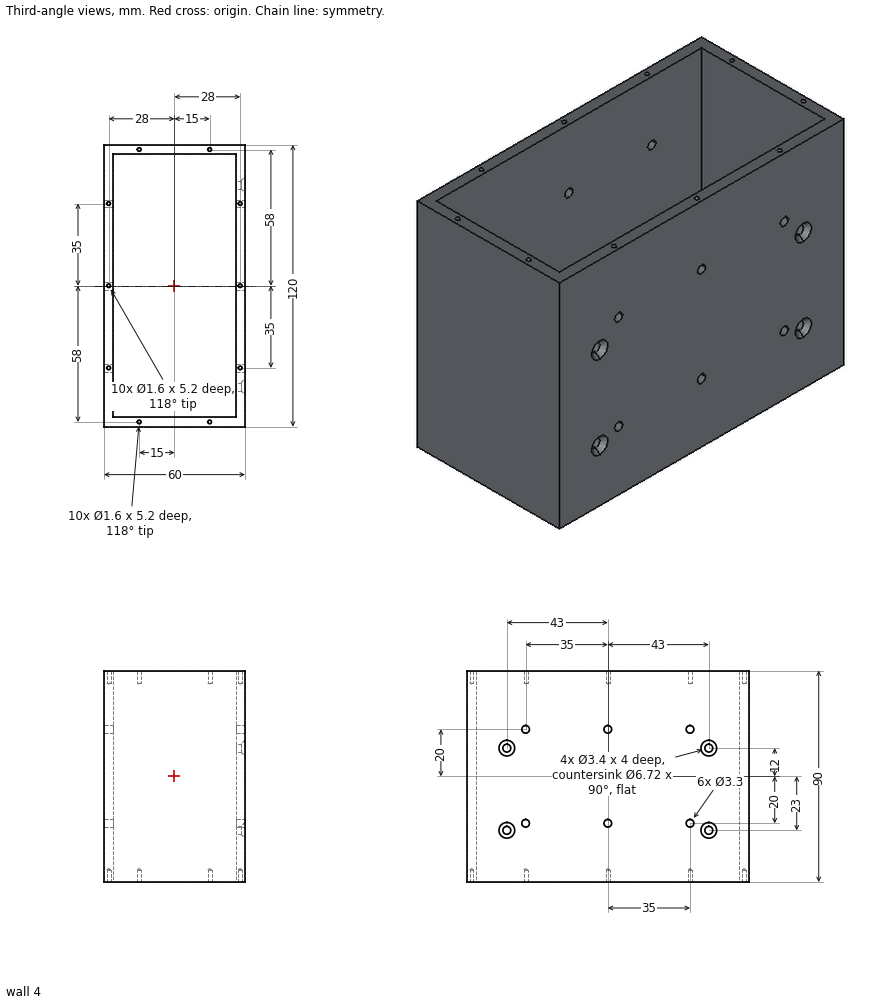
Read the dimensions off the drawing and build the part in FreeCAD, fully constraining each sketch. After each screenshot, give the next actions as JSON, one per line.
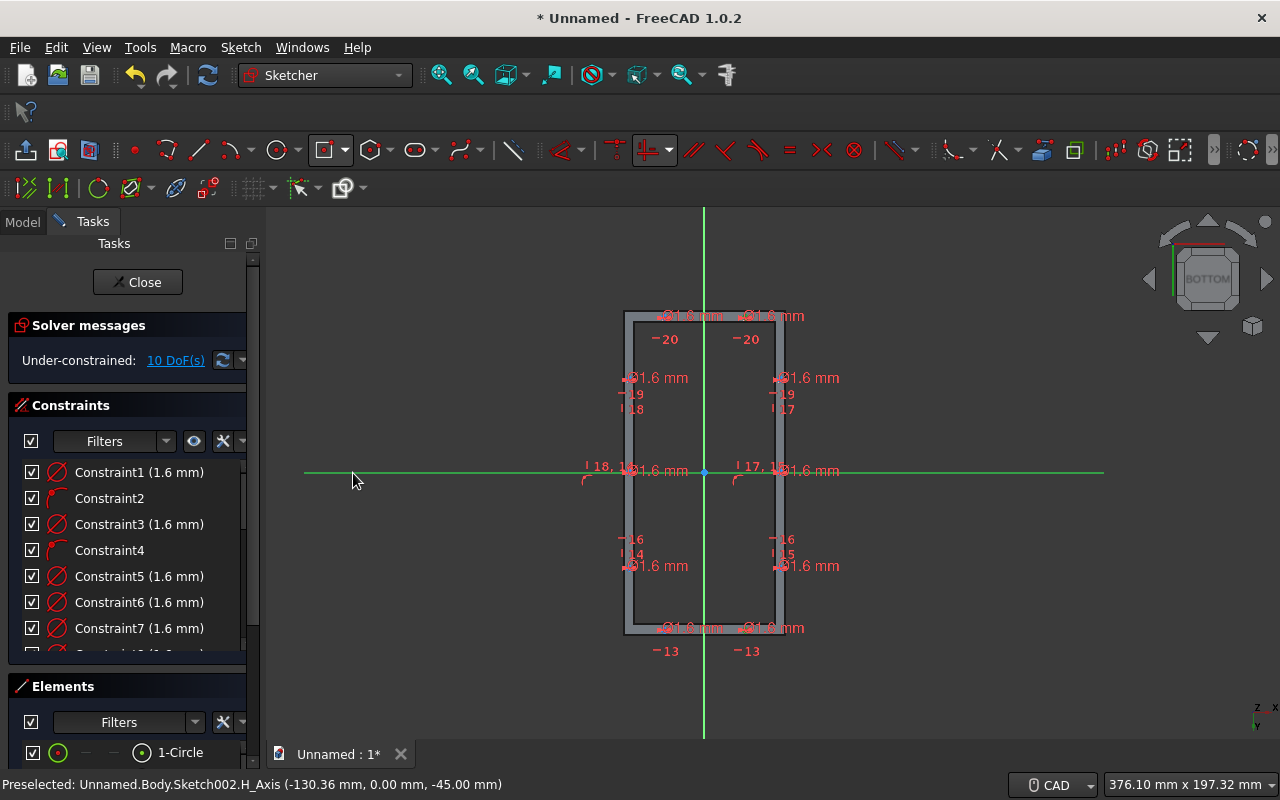
{"action": "left_click", "coordinate": [822, 150]}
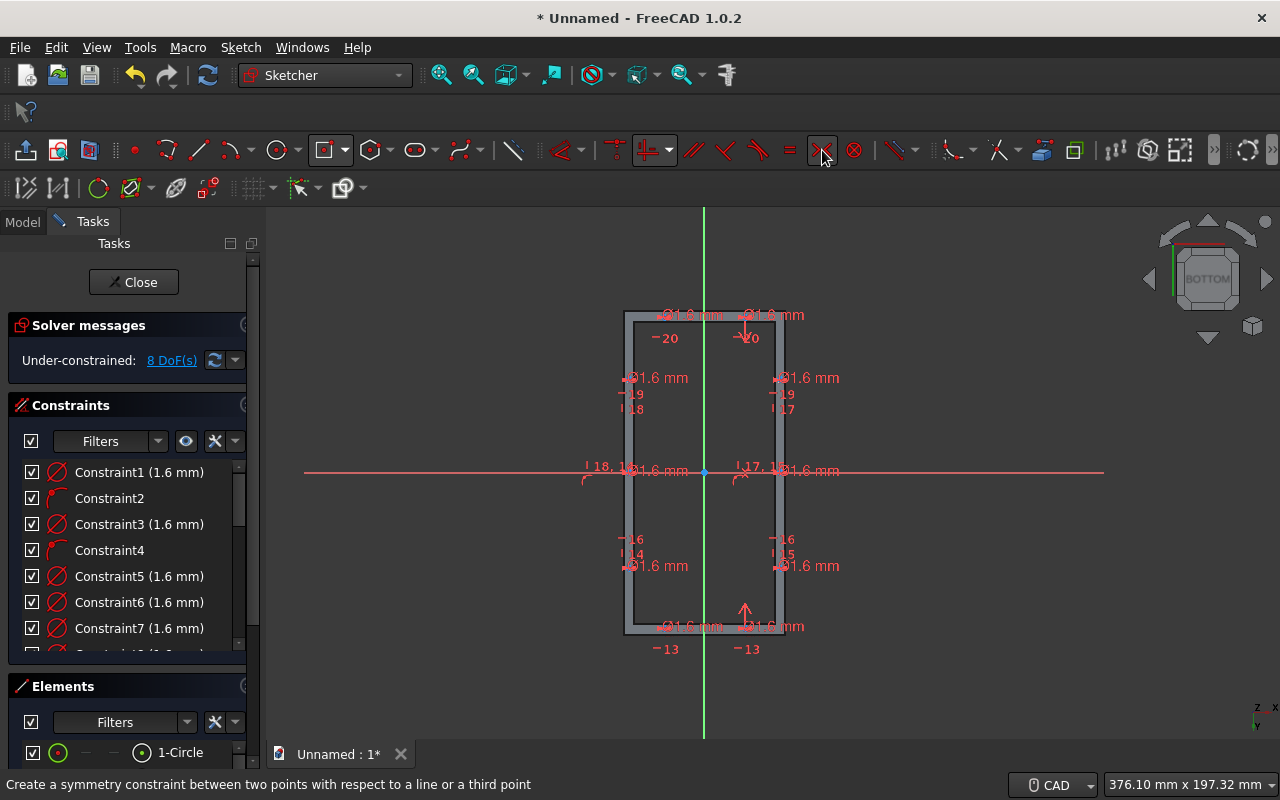
{"action": "left_click", "coordinate": [560, 150]}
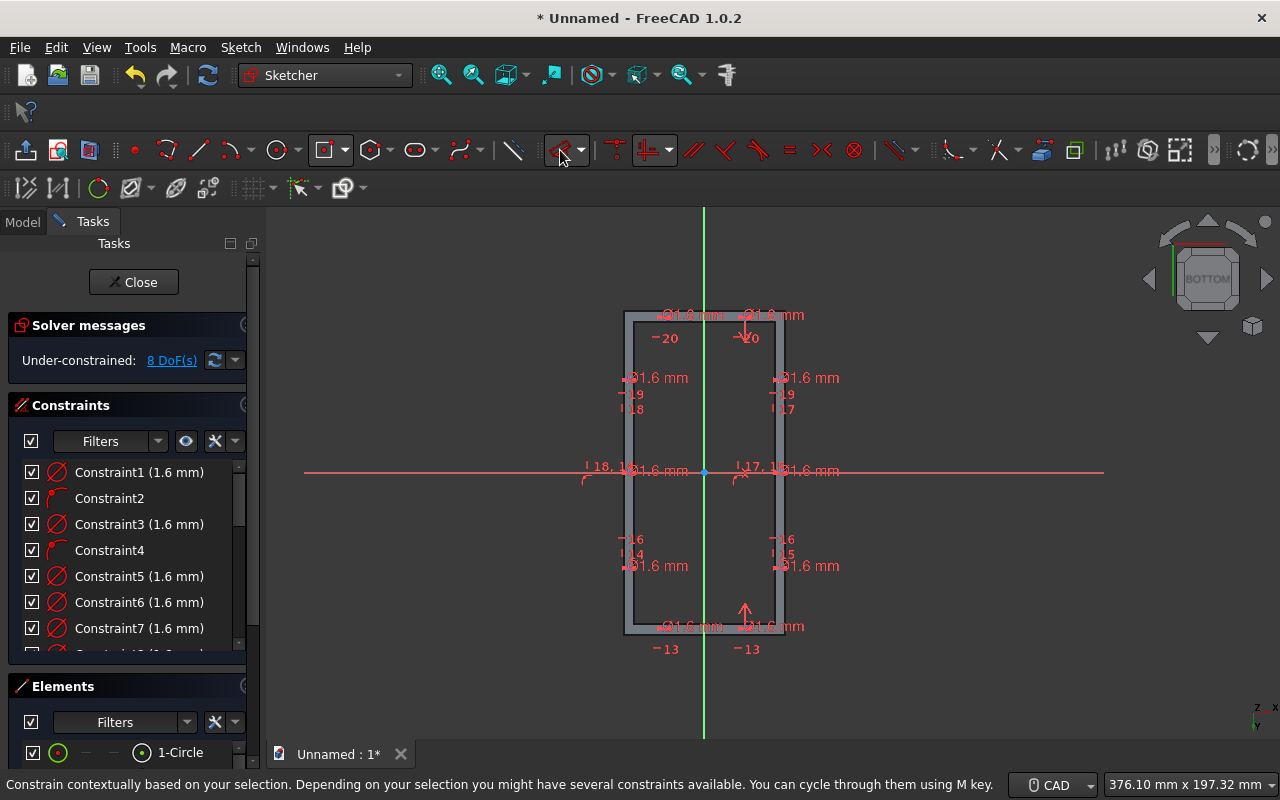
{"action": "left_click", "coordinate": [629, 473]}
{"action": "left_click", "coordinate": [667, 507]}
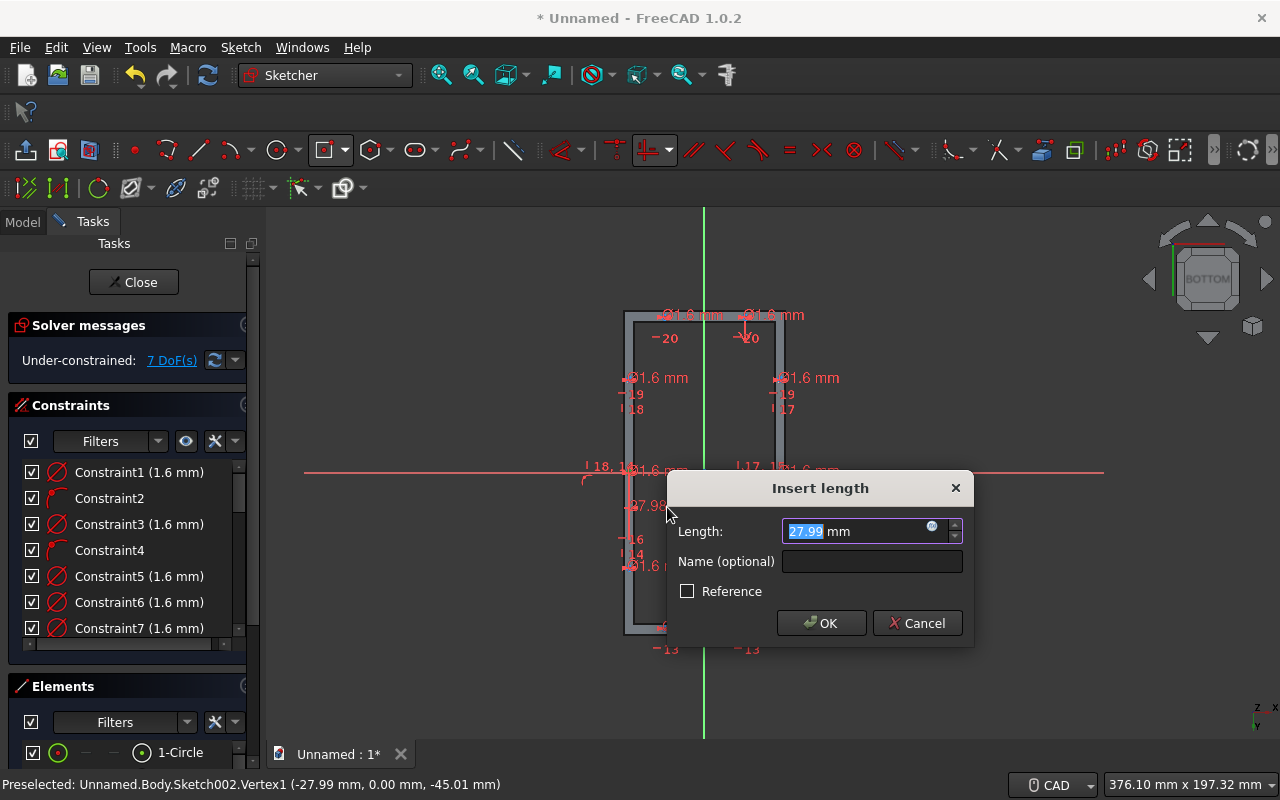
{"action": "type", "text": "28"}
{"action": "key", "text": "Return"}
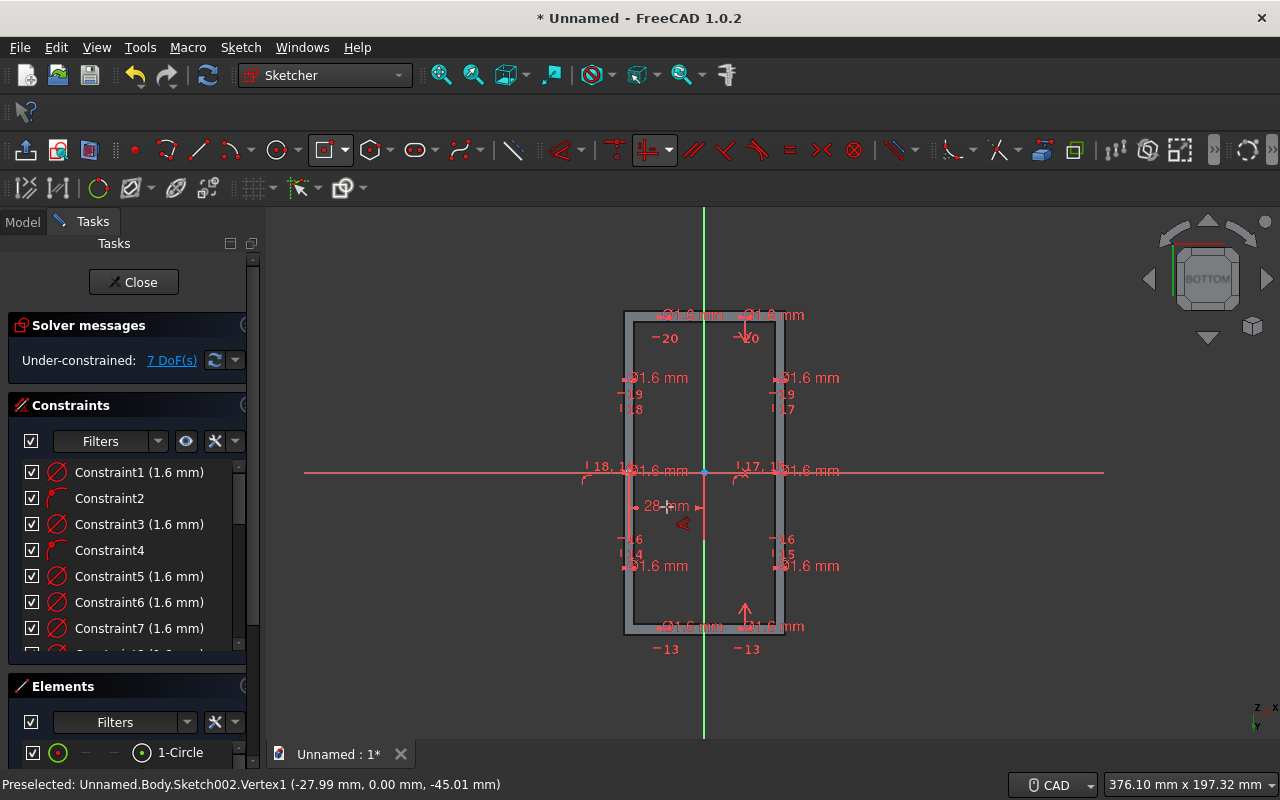
{"action": "left_click", "coordinate": [780, 473]}
{"action": "left_click", "coordinate": [742, 507]}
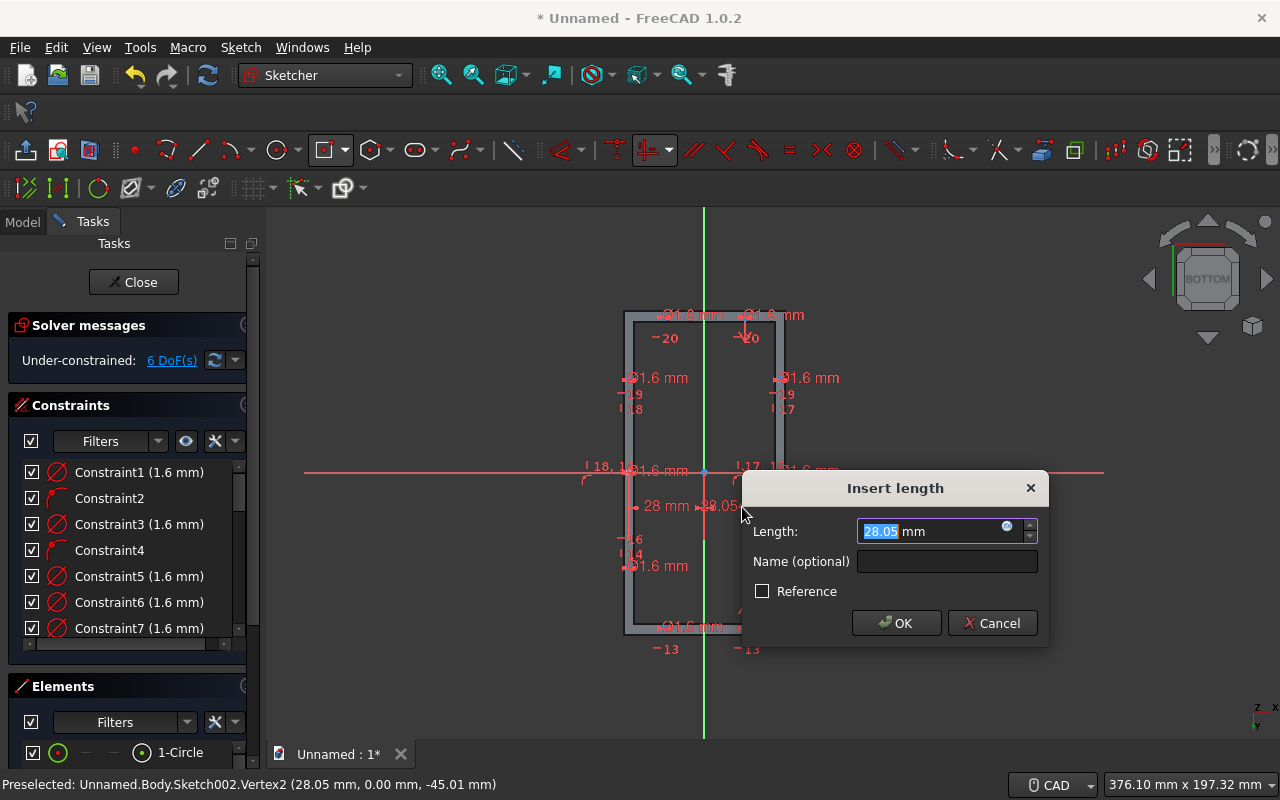
{"action": "type", "text": "28"}
{"action": "key", "text": "Return"}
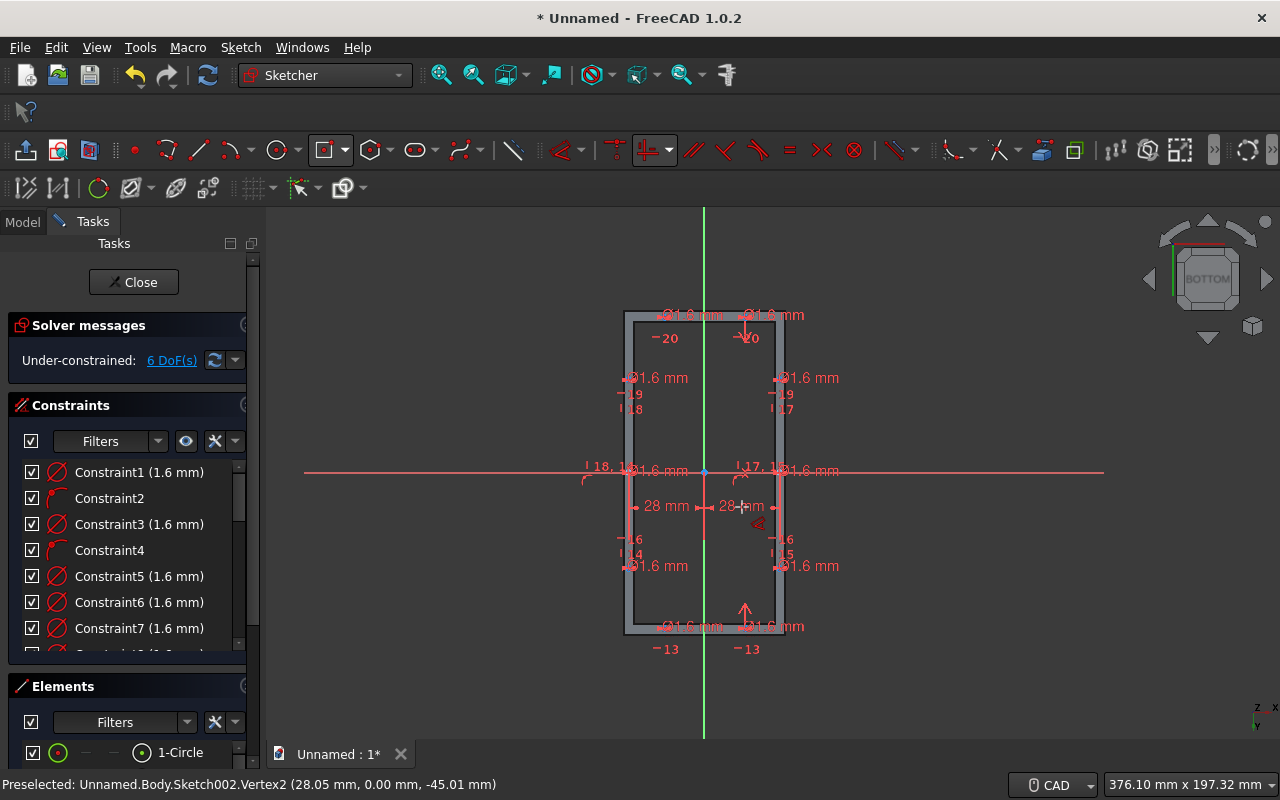
{"action": "left_click", "coordinate": [745, 629]}
{"action": "left_click", "coordinate": [725, 663]}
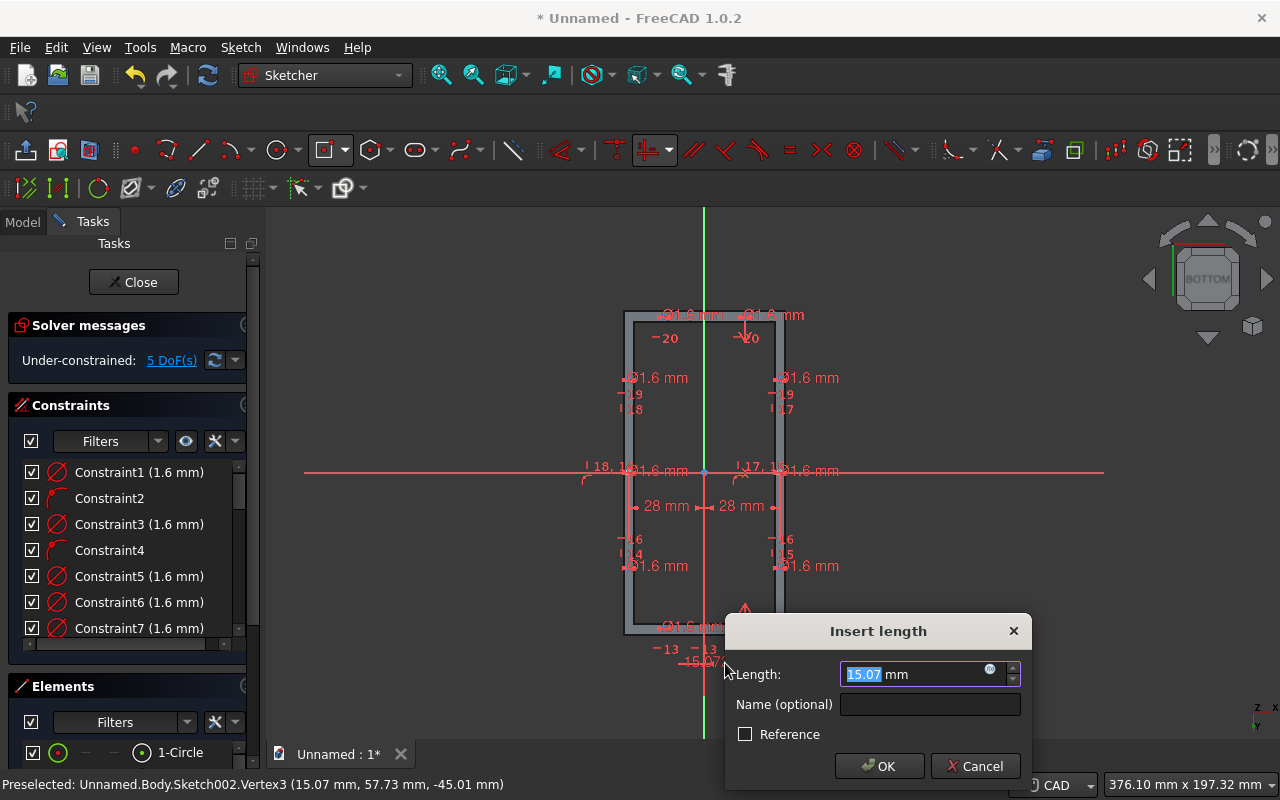
{"action": "type", "text": "15"}
{"action": "key", "text": "Return"}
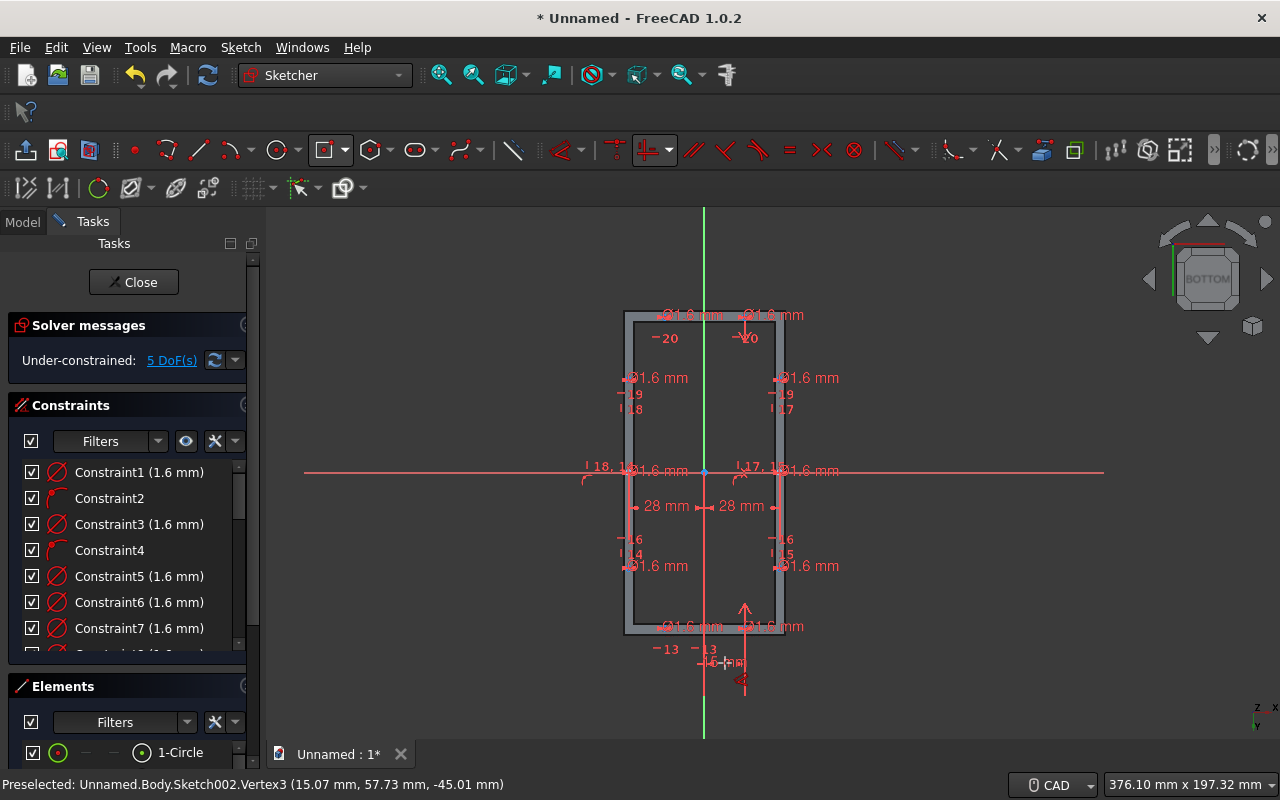
{"action": "left_click", "coordinate": [745, 629]}
{"action": "left_click", "coordinate": [779, 551]}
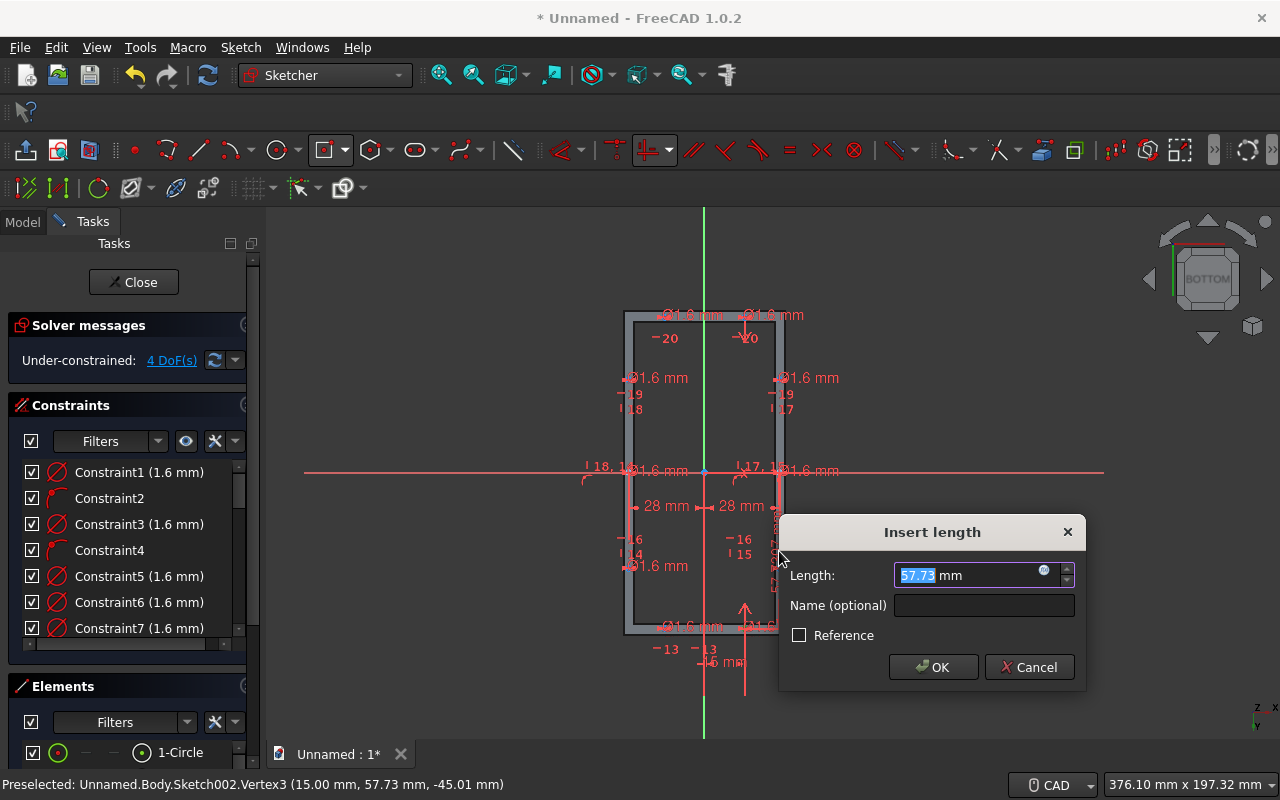
{"action": "type", "text": "58"}
{"action": "key", "text": "Return"}